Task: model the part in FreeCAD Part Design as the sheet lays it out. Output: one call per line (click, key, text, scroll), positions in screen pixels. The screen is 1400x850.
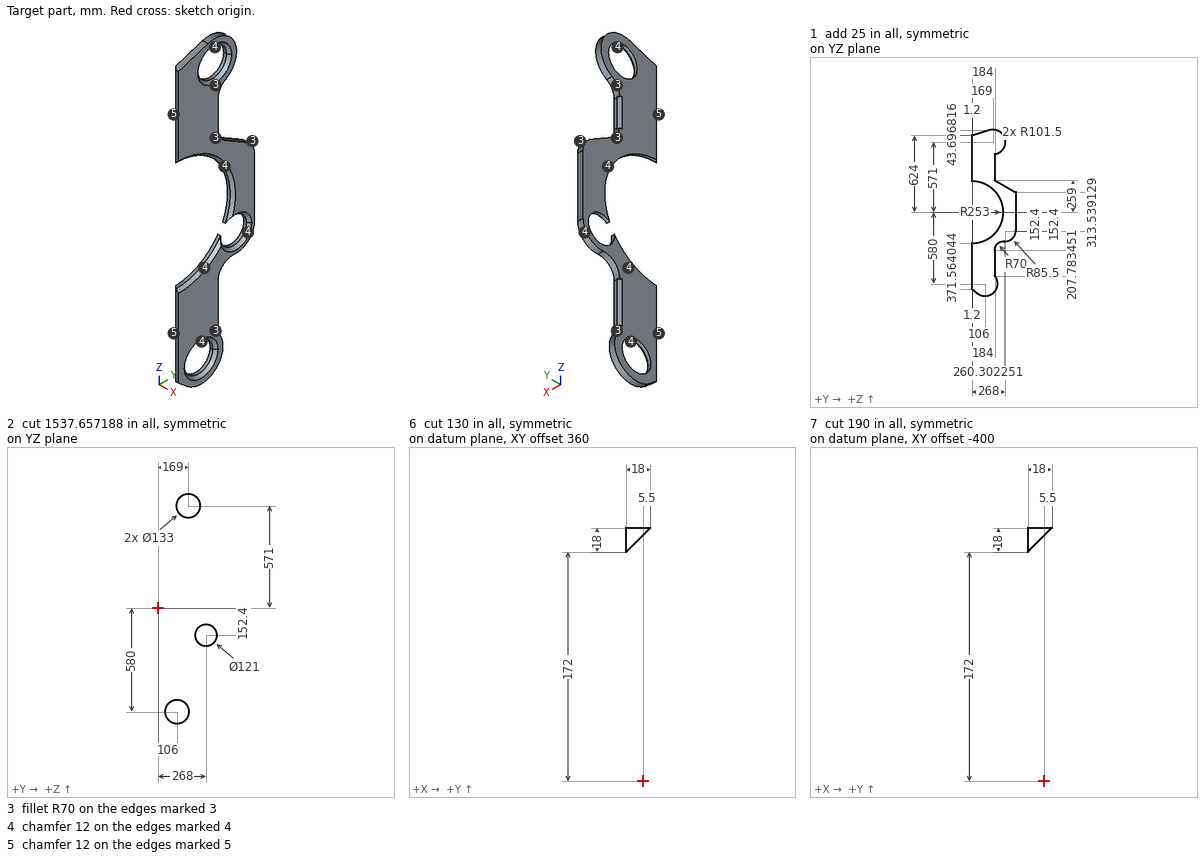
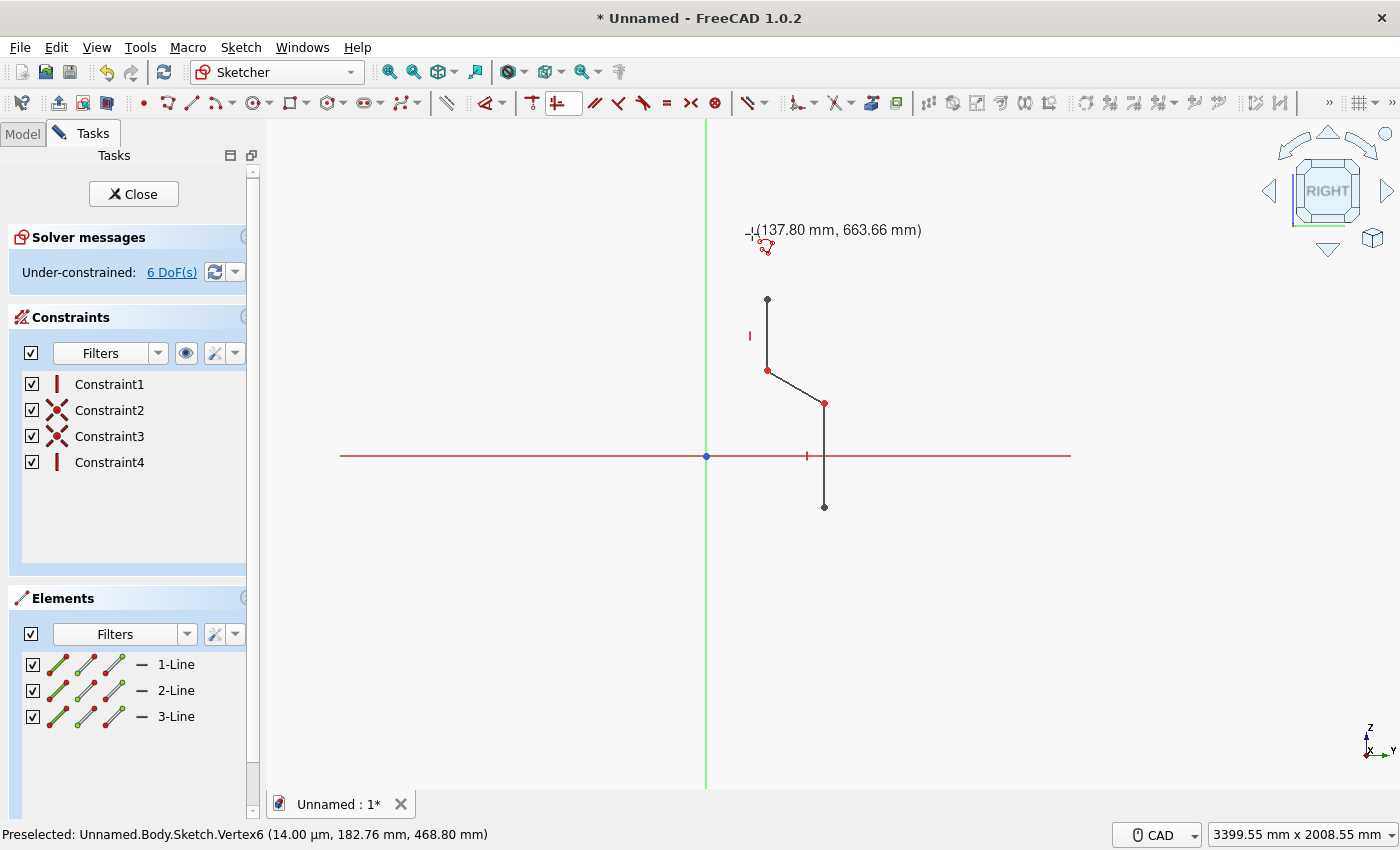
scroll(706, 248, up, 19)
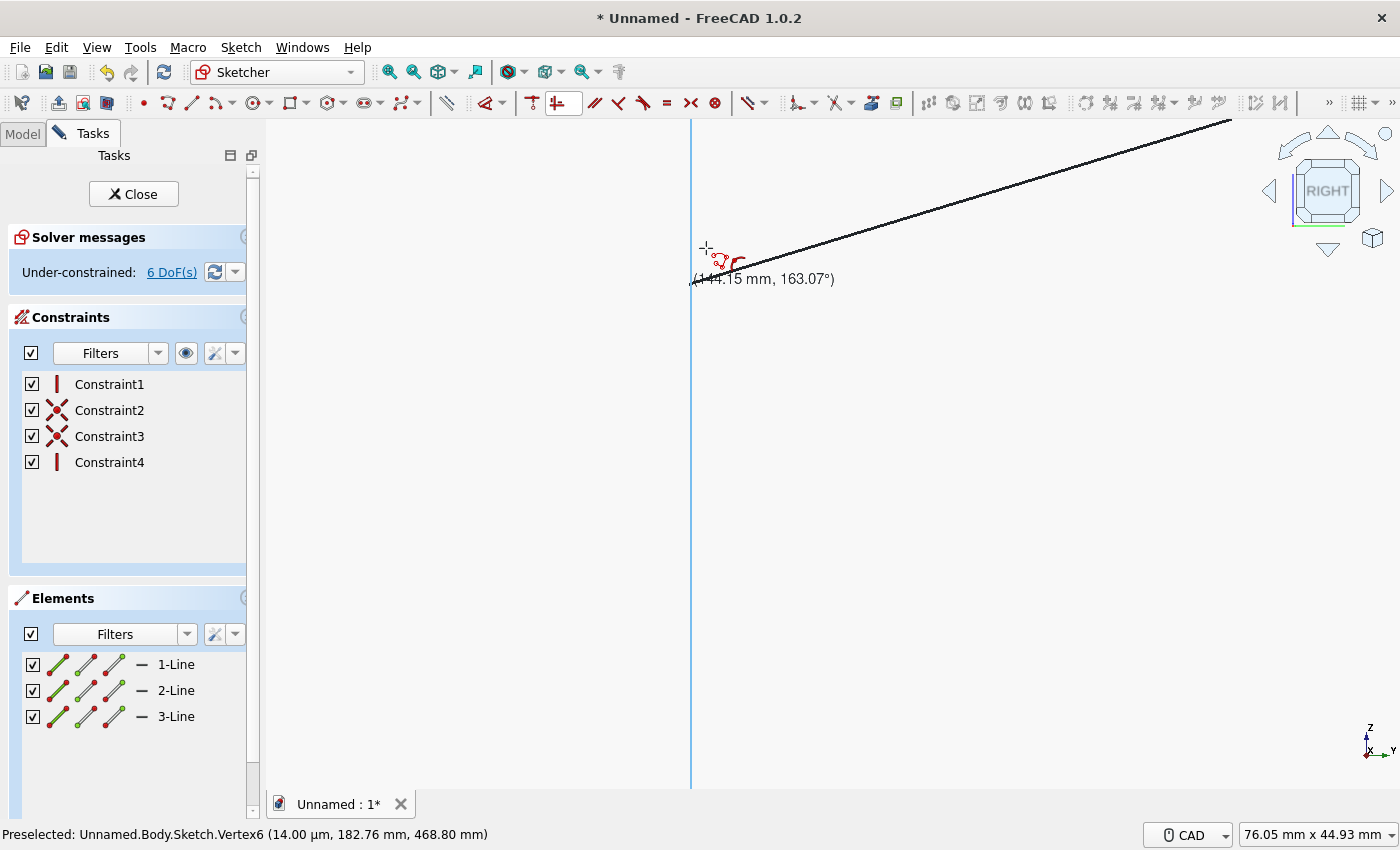
click(708, 250)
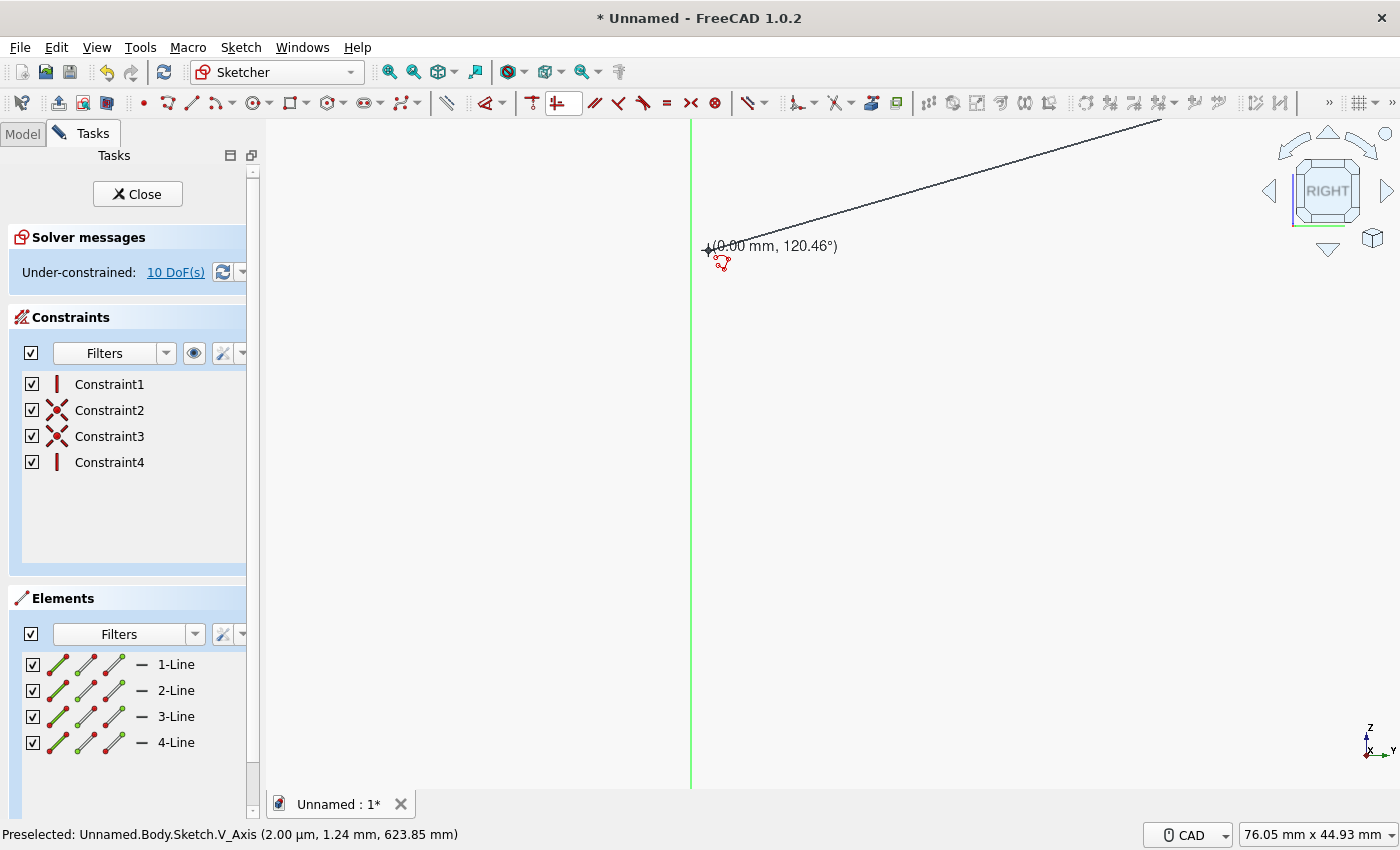
scroll(693, 200, down, 18)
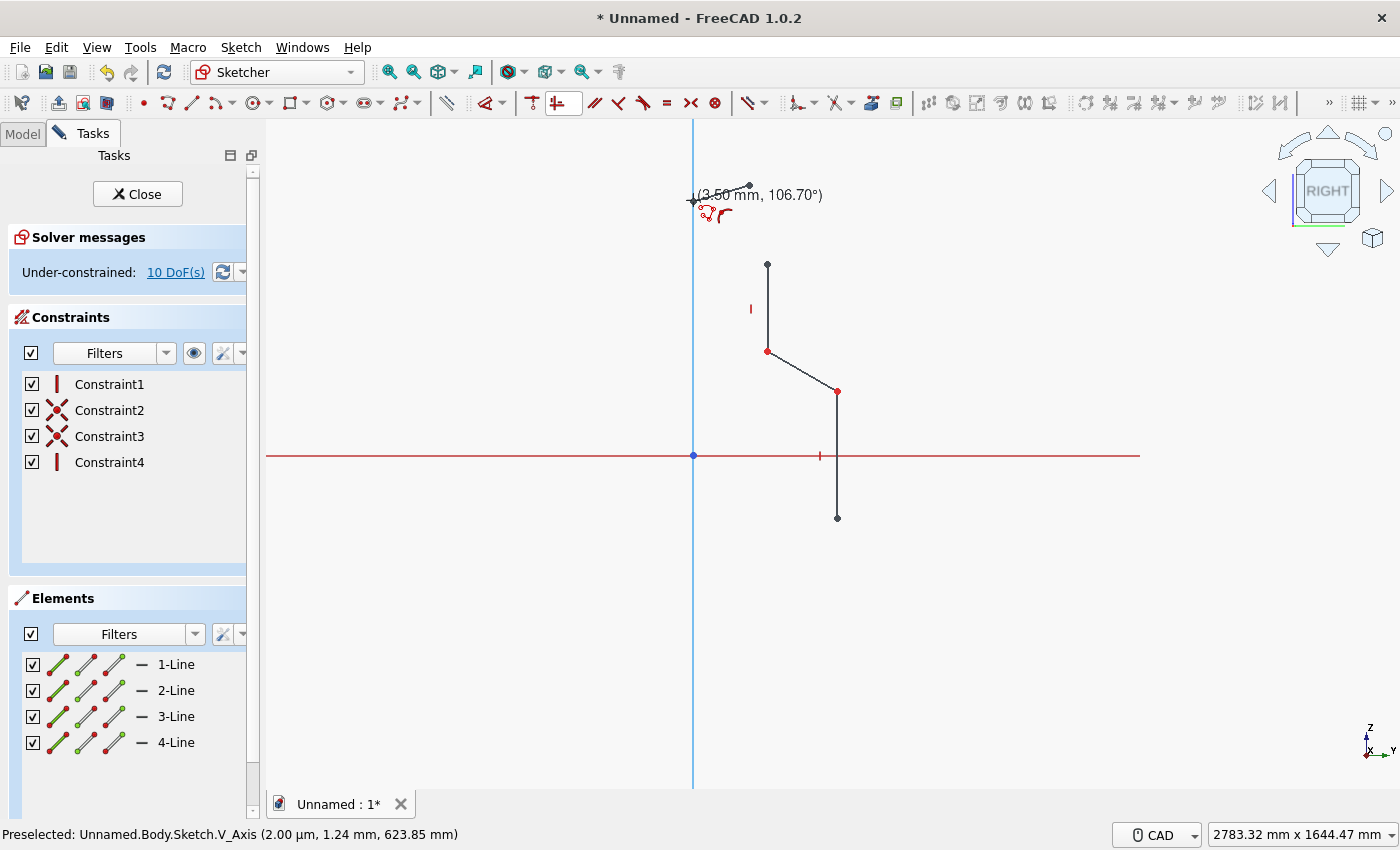
scroll(694, 353, up, 18)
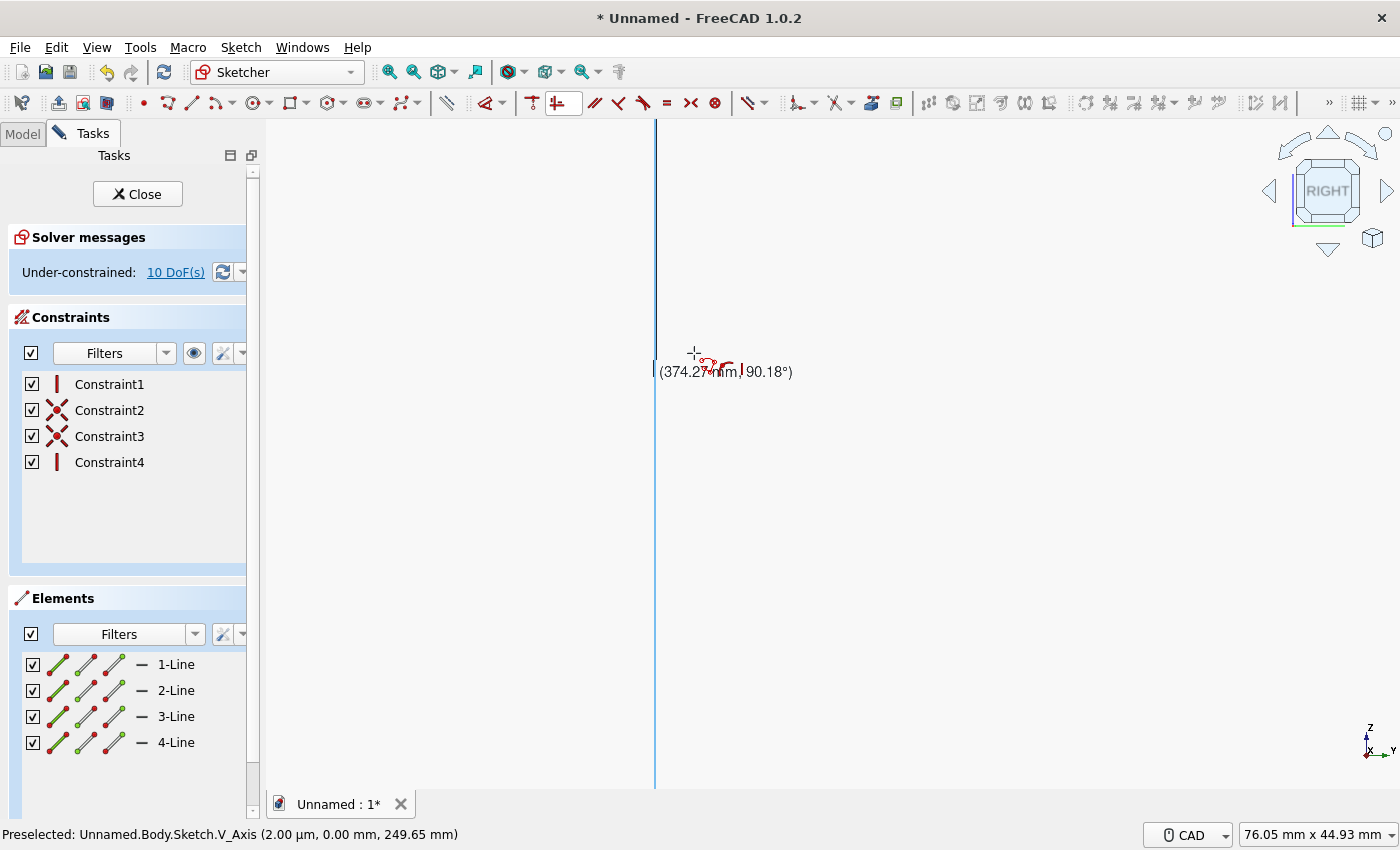
click(672, 327)
right_click(672, 327)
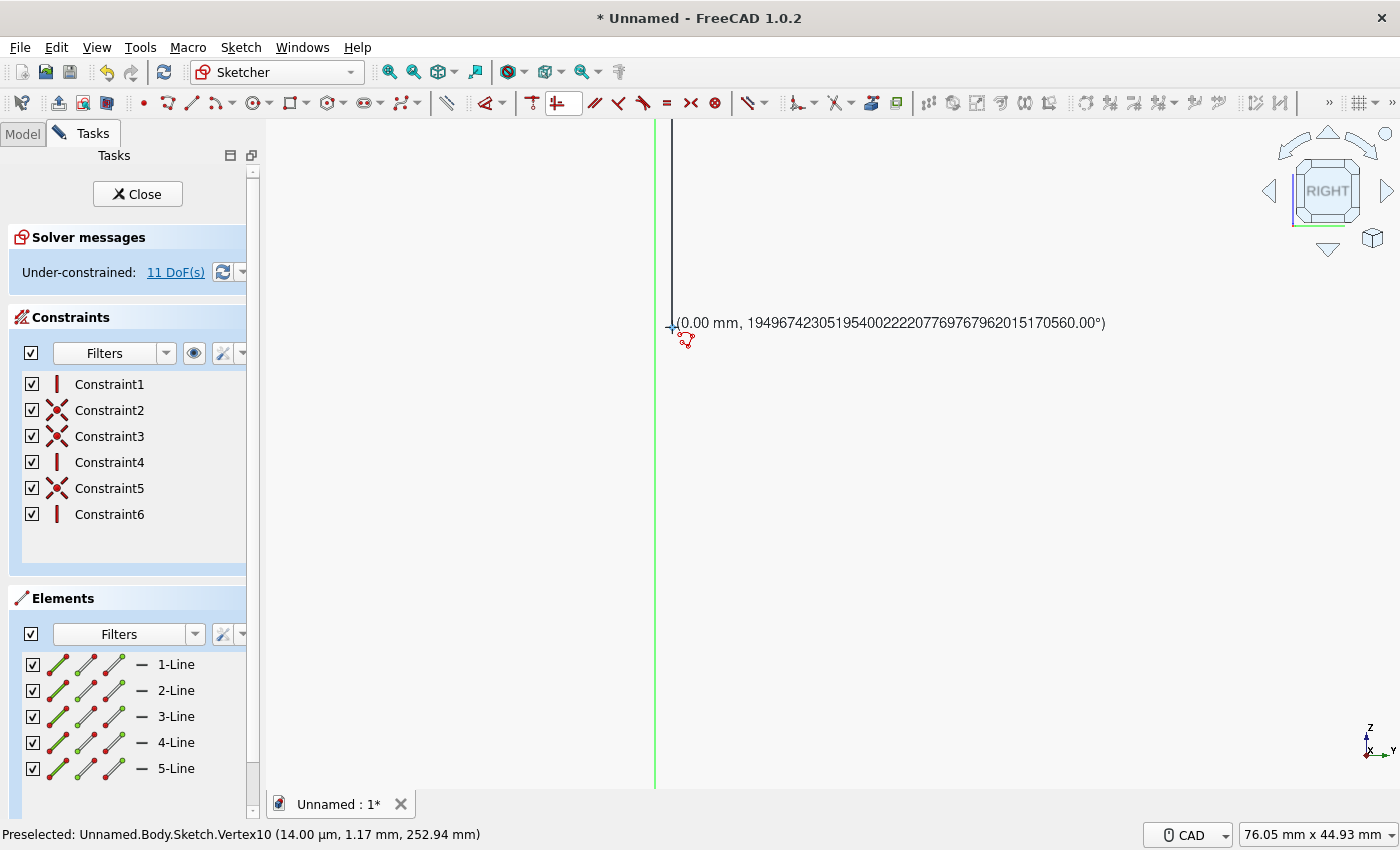
scroll(694, 354, down, 18)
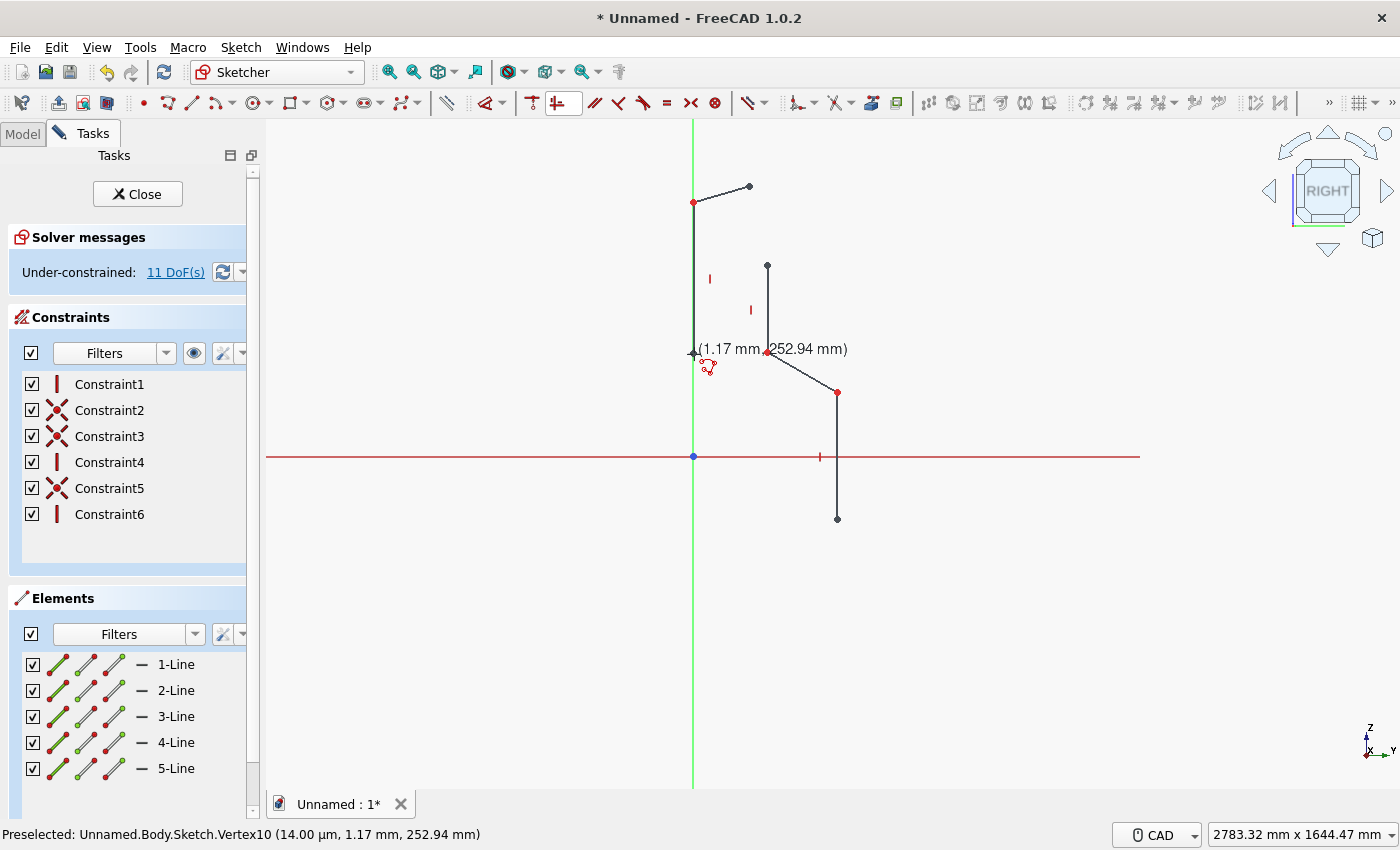
scroll(694, 560, up, 18)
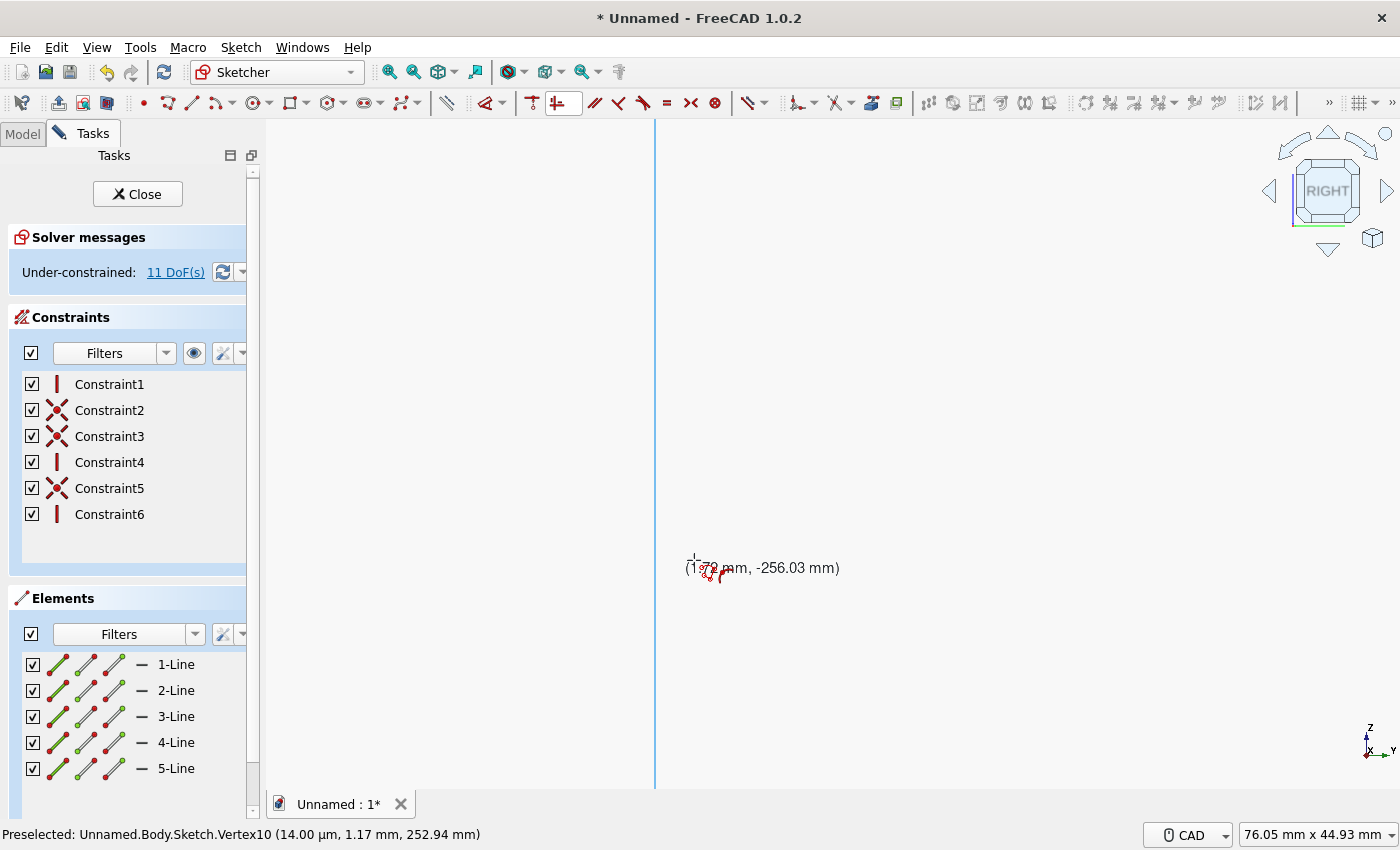
click(673, 528)